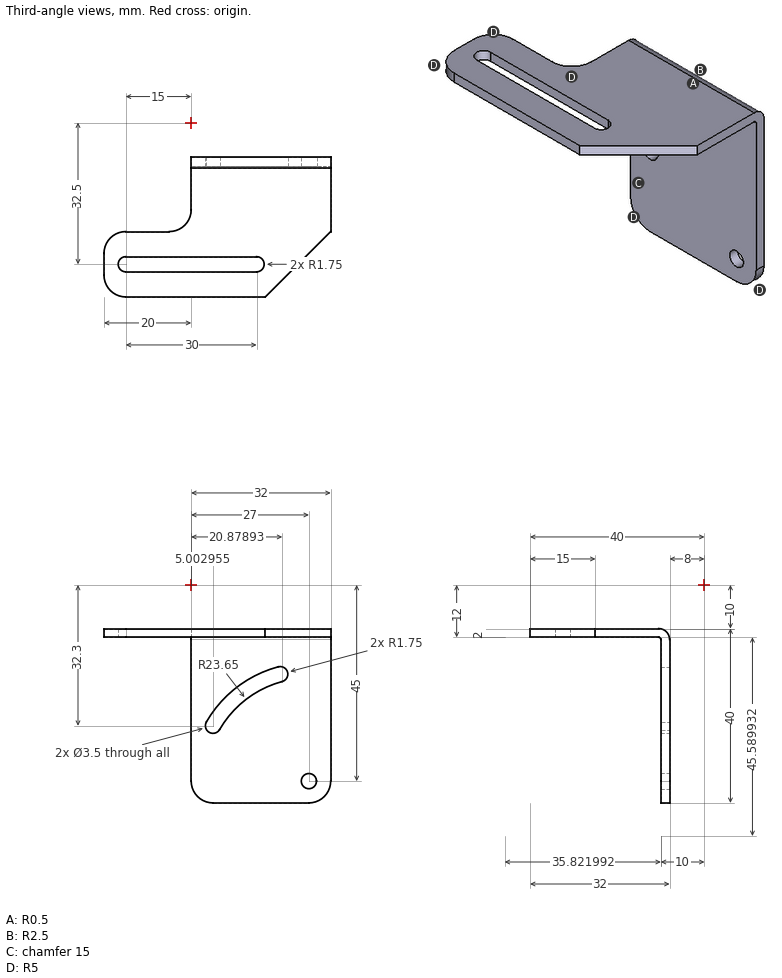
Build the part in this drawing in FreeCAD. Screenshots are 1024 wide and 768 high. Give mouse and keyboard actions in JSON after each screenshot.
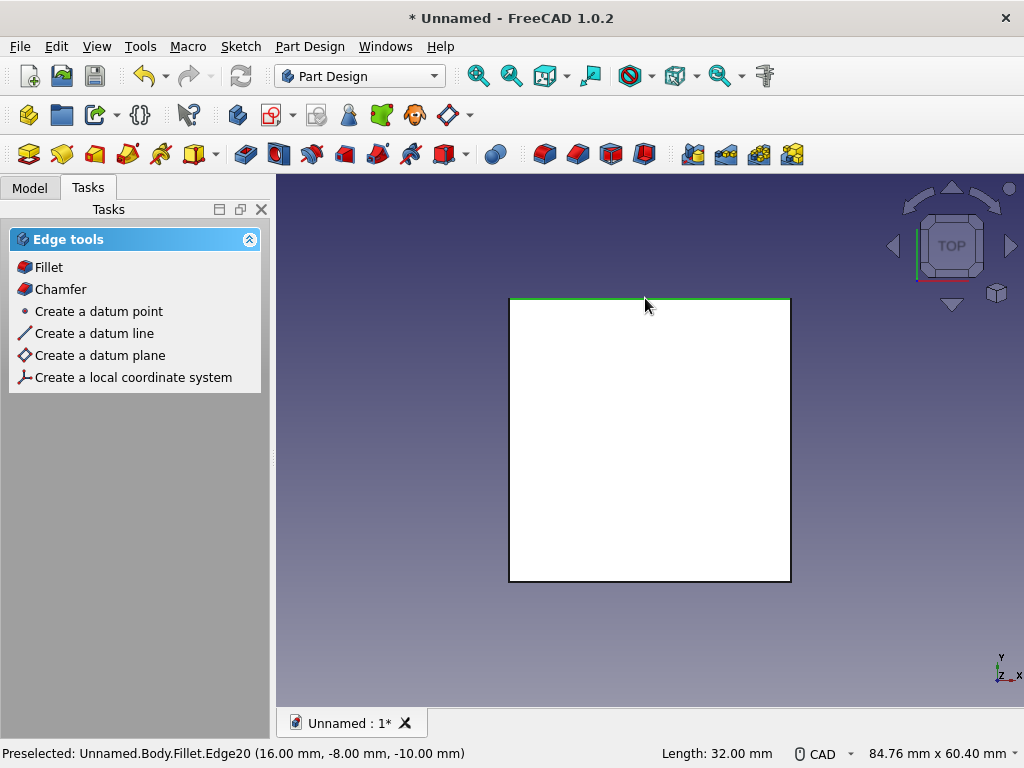
{"action": "left_click", "coordinate": [545, 154]}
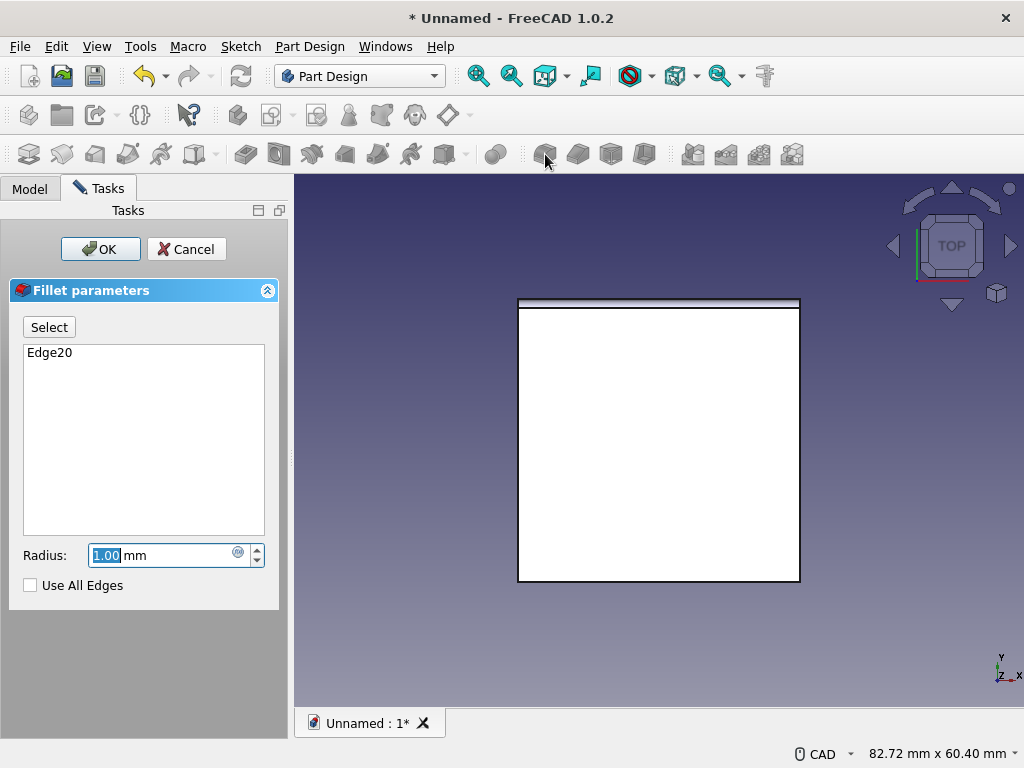
{"action": "type", "text": "2.5"}
{"action": "key", "text": "Tab"}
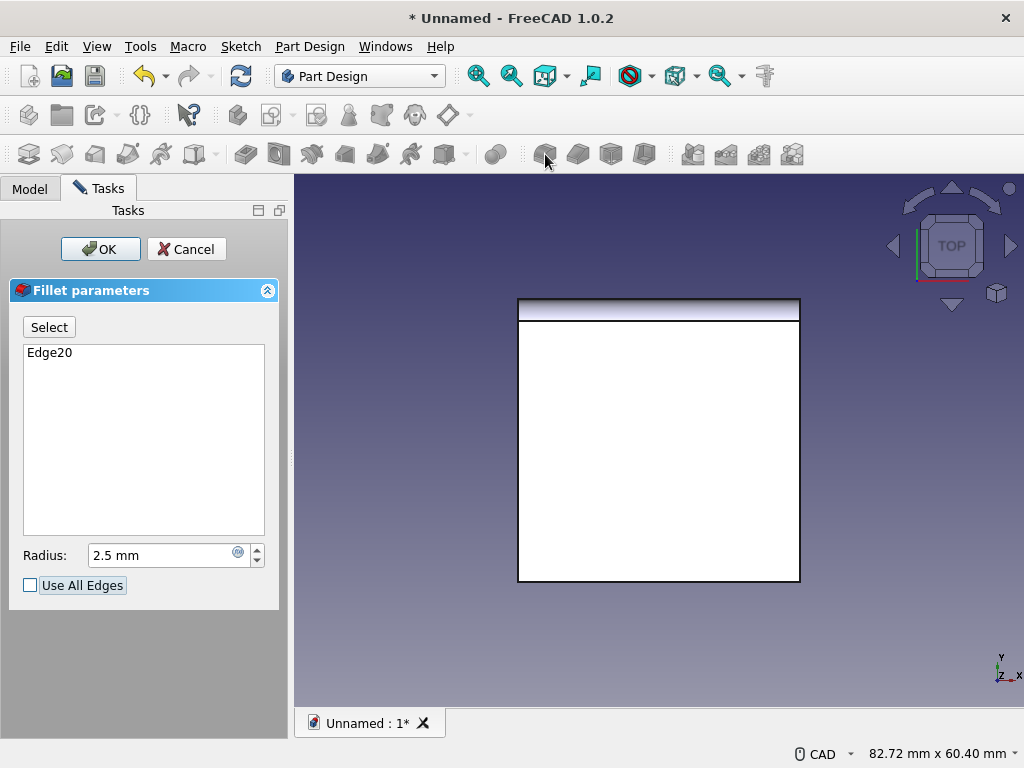
{"action": "left_click", "coordinate": [101, 249]}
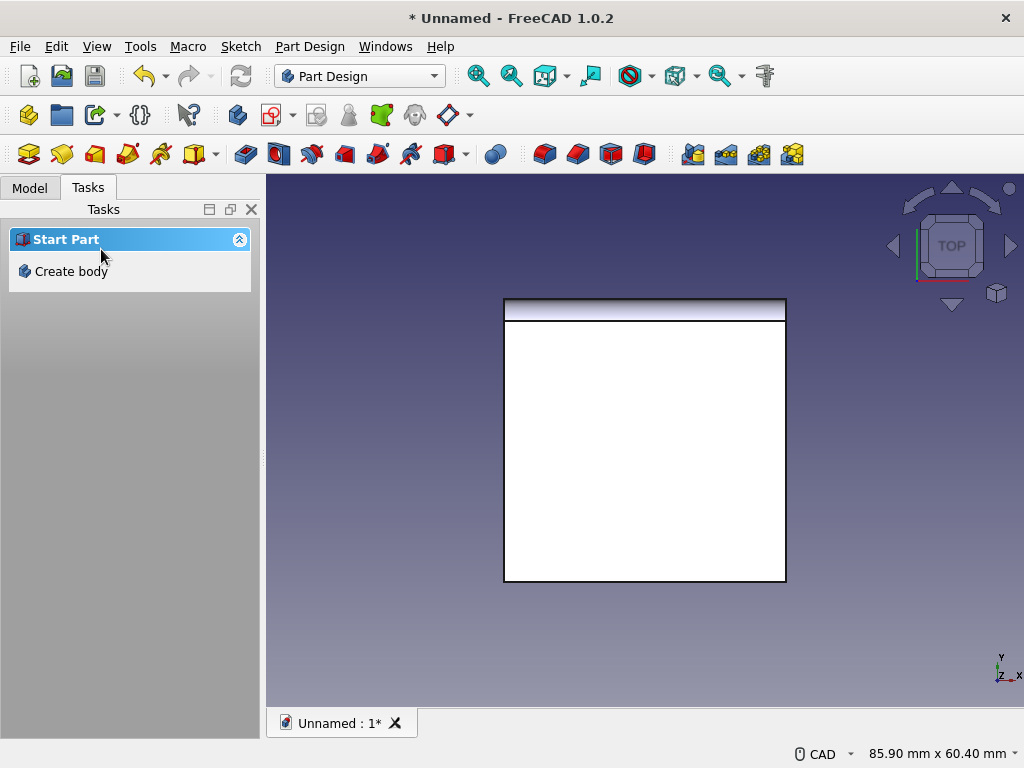
{"action": "key", "text": "4"}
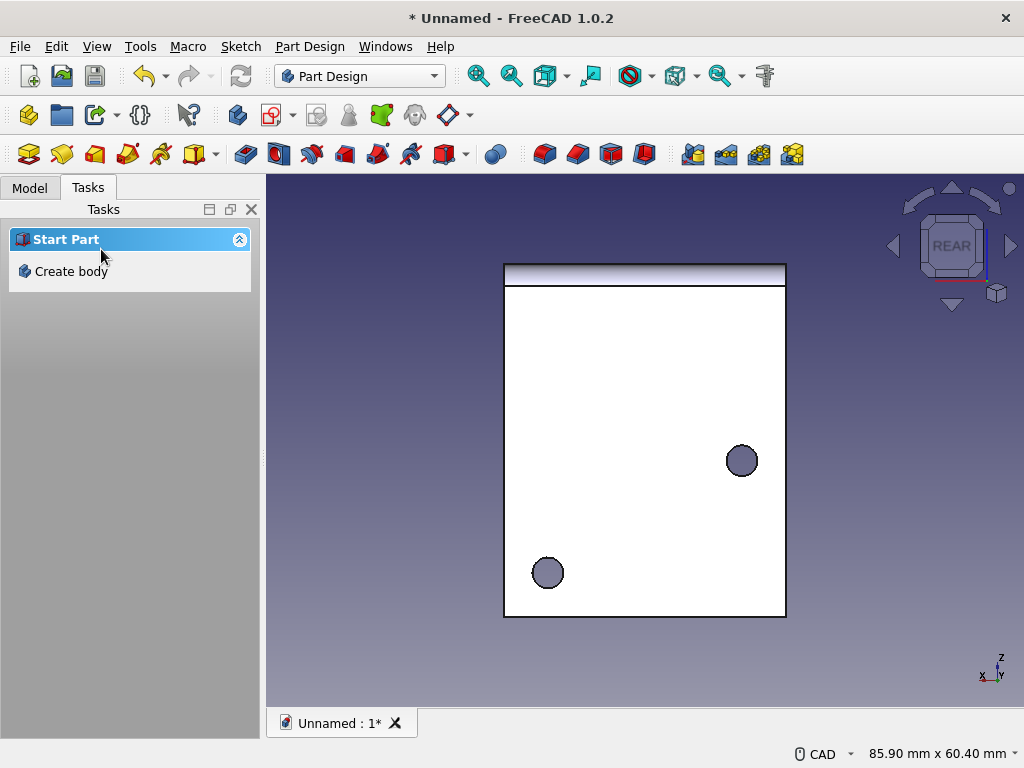
{"action": "left_click", "coordinate": [605, 403]}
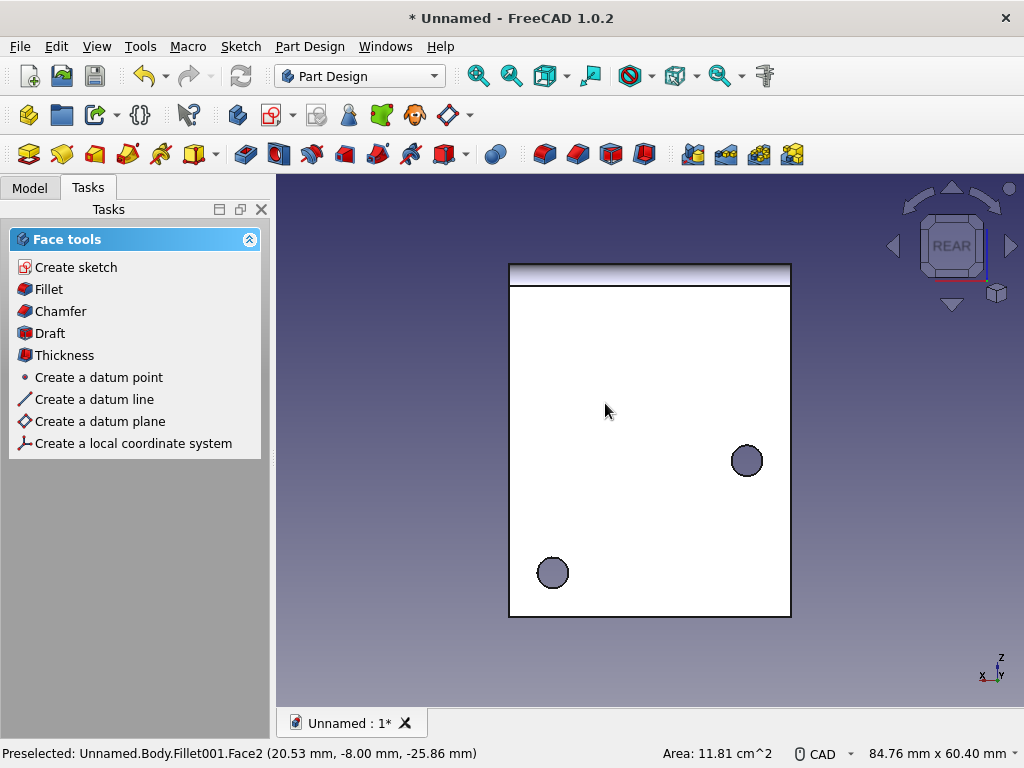
{"action": "left_click", "coordinate": [270, 116]}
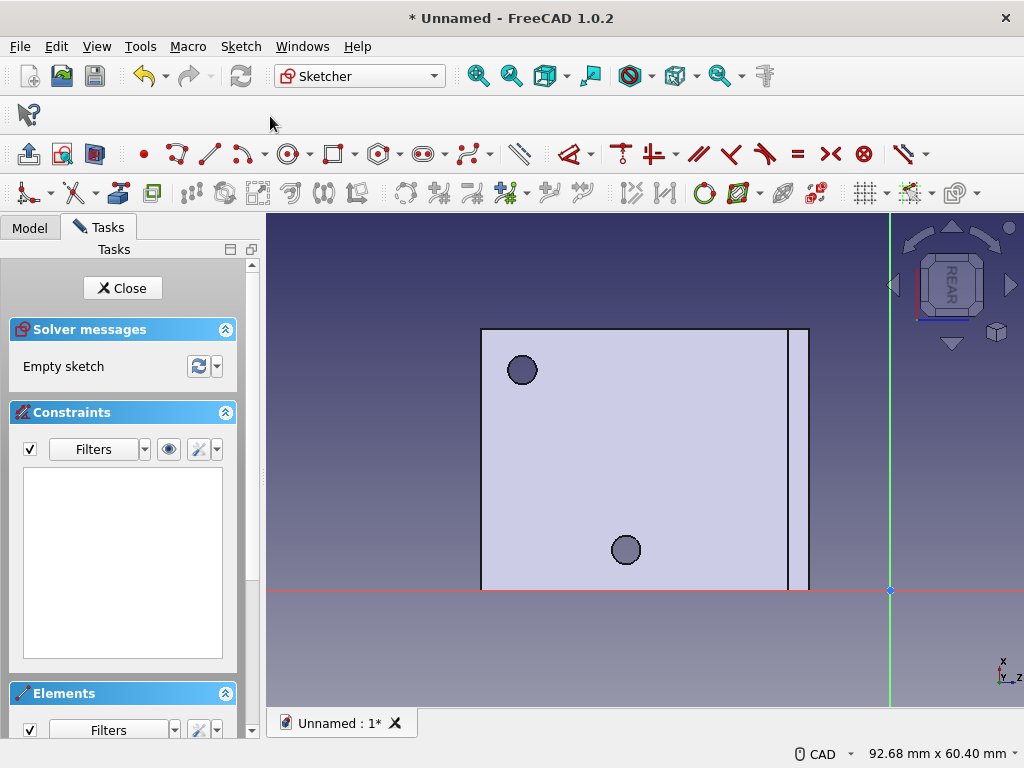
{"action": "scroll", "coordinate": [294, 277], "scroll_direction": "down", "scroll_amount": 1}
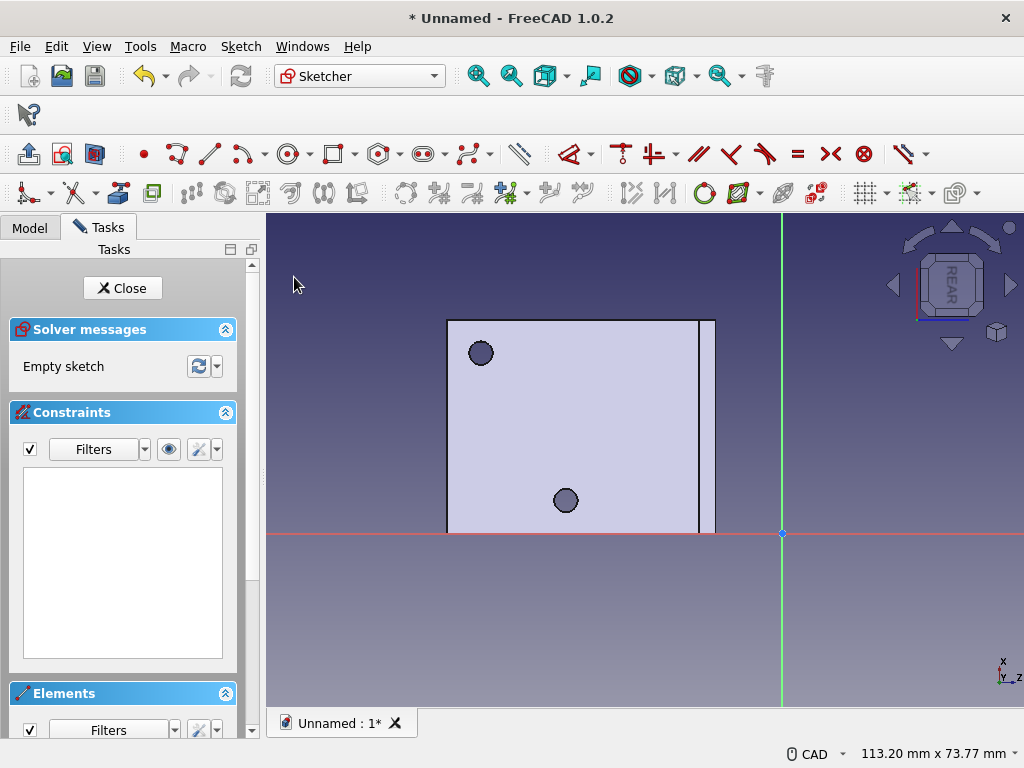
{"action": "scroll", "coordinate": [782, 460], "scroll_direction": "up", "scroll_amount": 3}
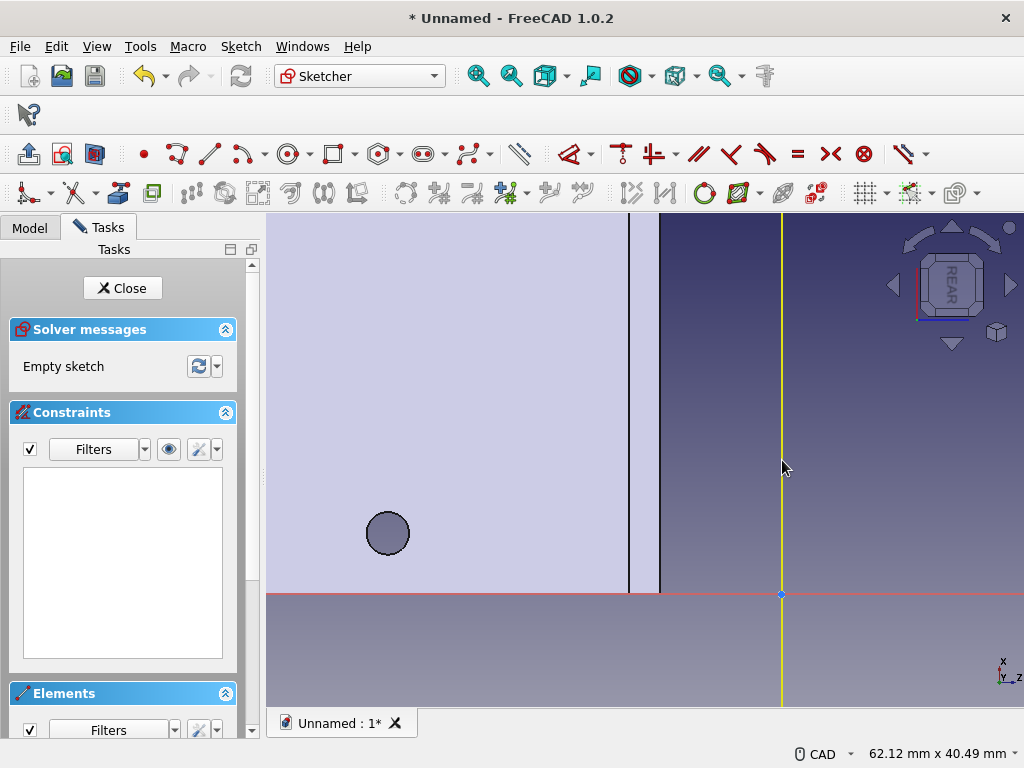
{"action": "key", "text": "g 3 a"}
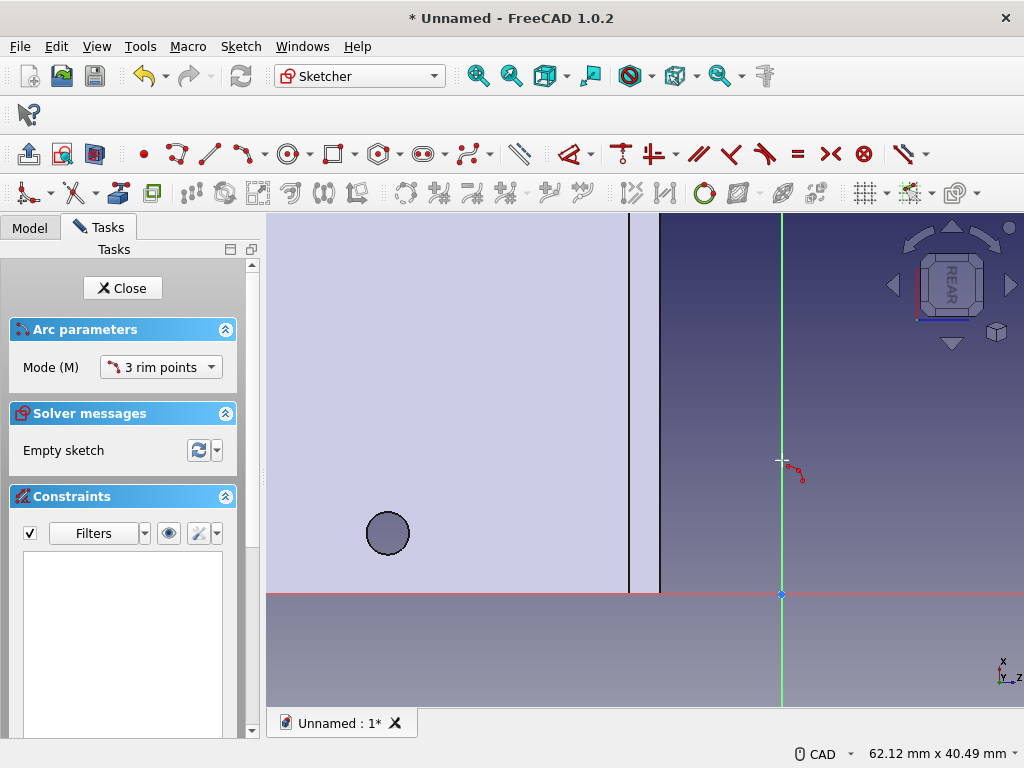
{"action": "left_click", "coordinate": [553, 351]}
{"action": "left_click", "coordinate": [512, 340]}
{"action": "left_click", "coordinate": [538, 325]}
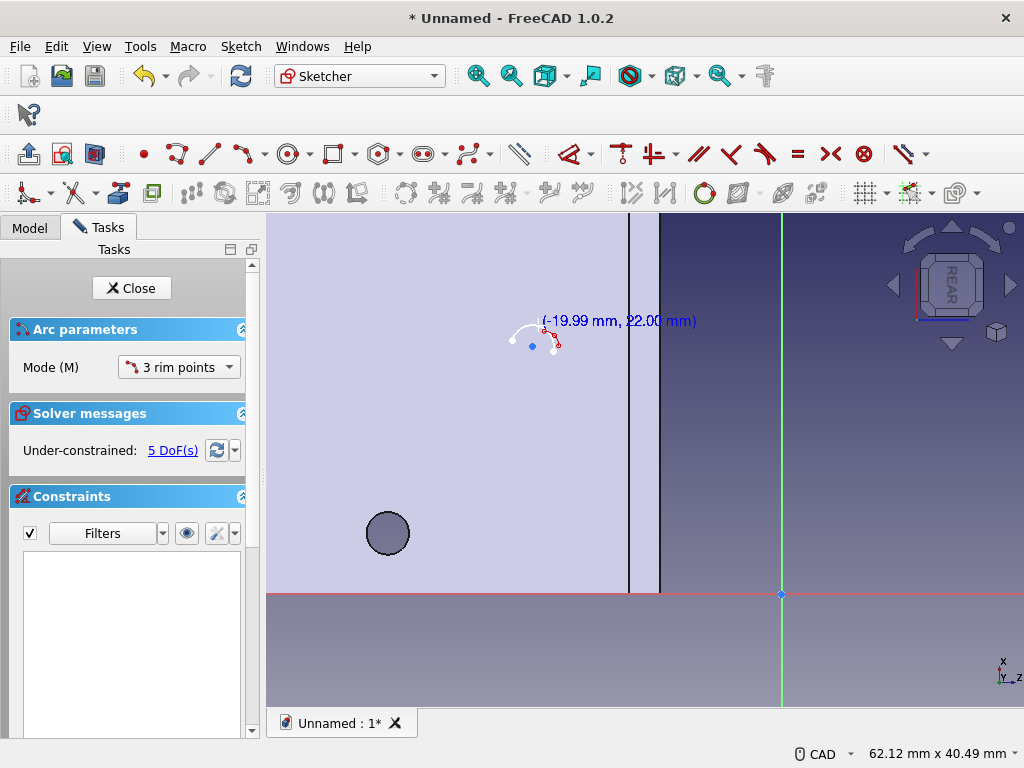
{"action": "left_click", "coordinate": [512, 341]}
{"action": "left_click", "coordinate": [377, 515]}
{"action": "left_click", "coordinate": [462, 441]}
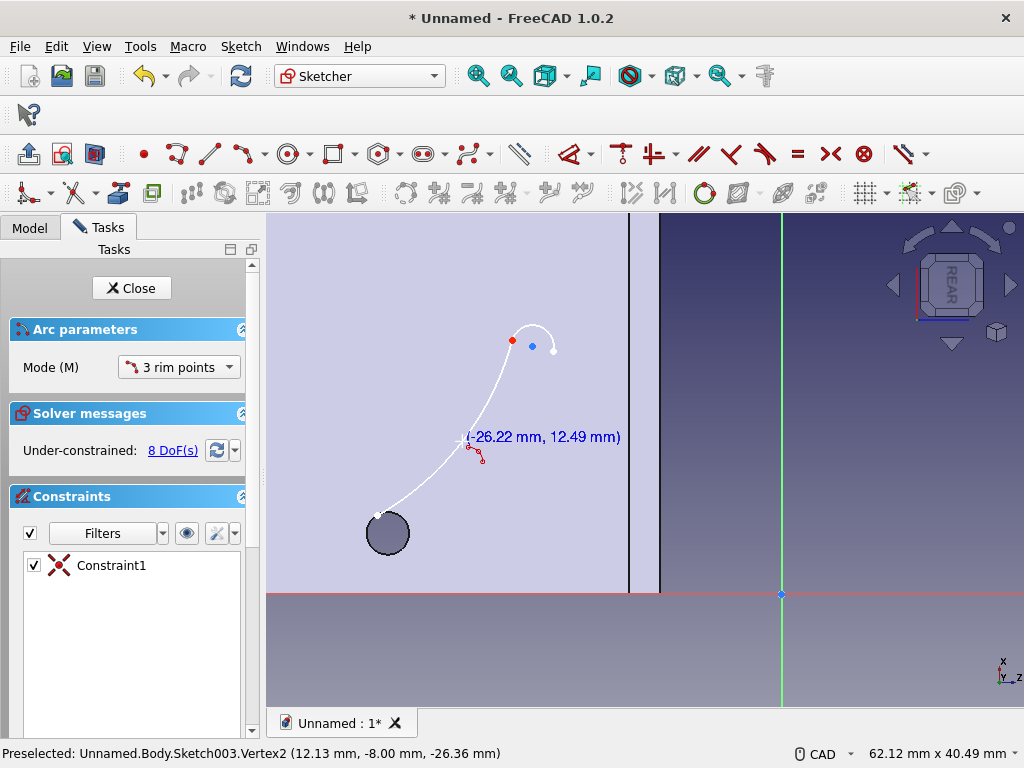
{"action": "left_click", "coordinate": [377, 516]}
{"action": "left_click", "coordinate": [399, 552]}
{"action": "left_click", "coordinate": [369, 544]}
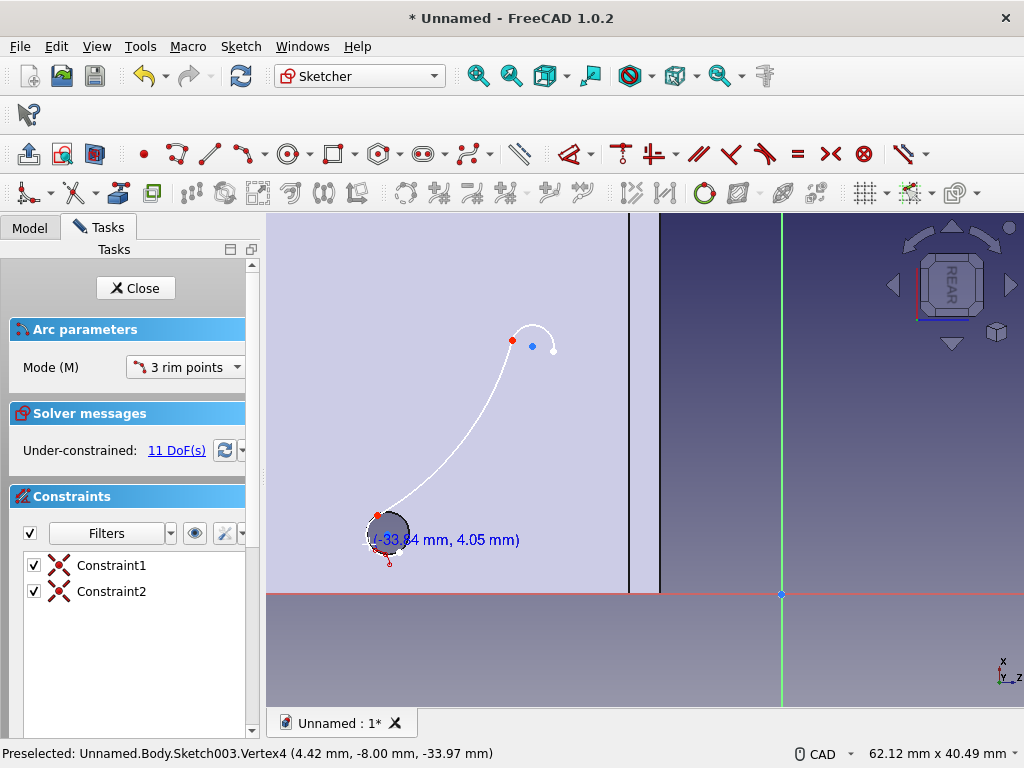
{"action": "left_click", "coordinate": [399, 553]}
{"action": "left_click", "coordinate": [553, 352]}
{"action": "left_click", "coordinate": [496, 467]}
{"action": "key", "text": "Escape"}